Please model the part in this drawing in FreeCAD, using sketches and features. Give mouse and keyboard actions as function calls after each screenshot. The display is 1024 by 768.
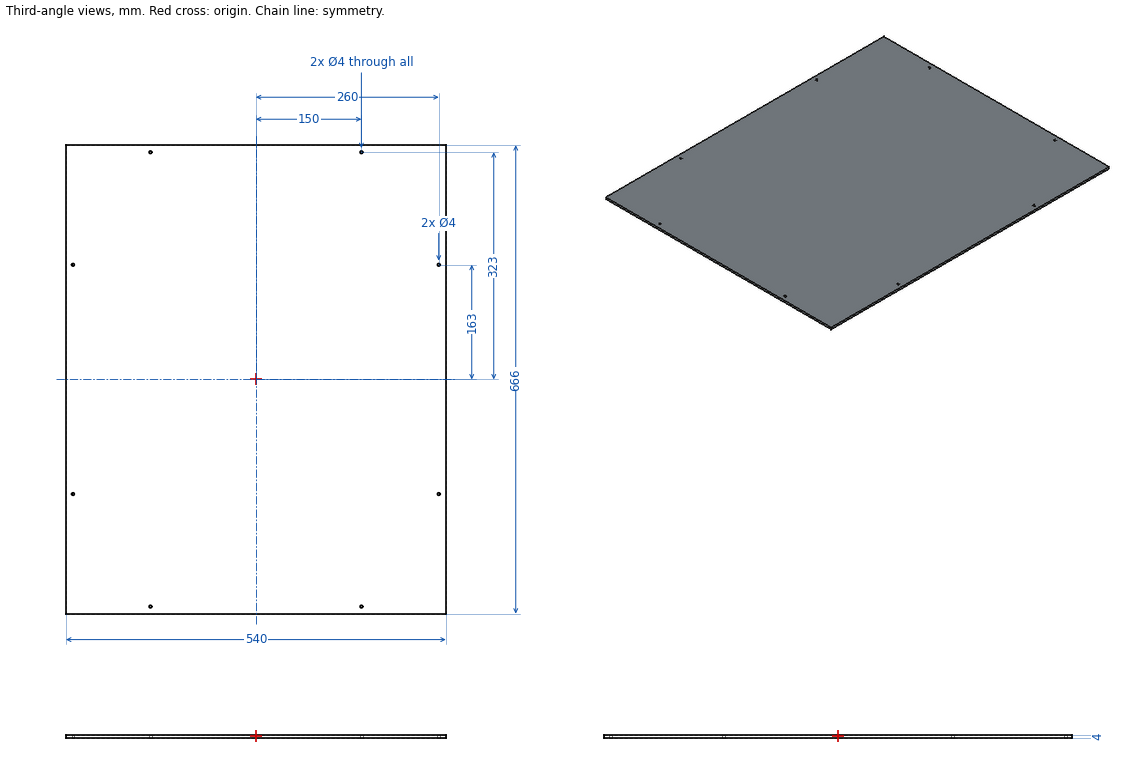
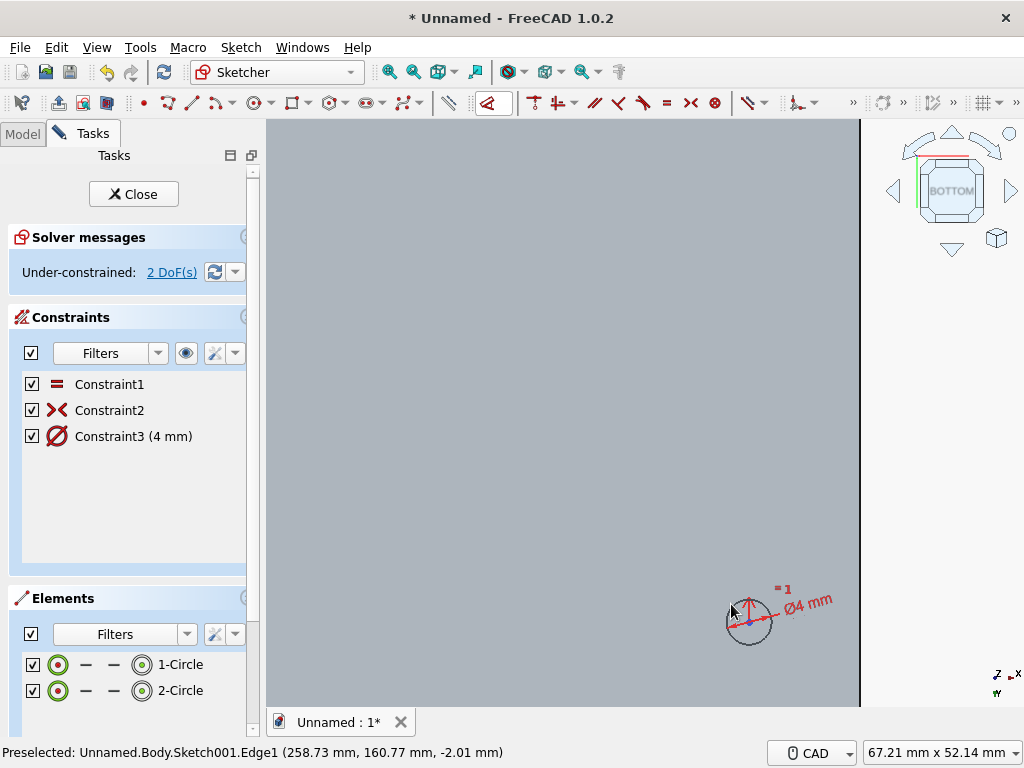
scroll(736, 615, down, 11)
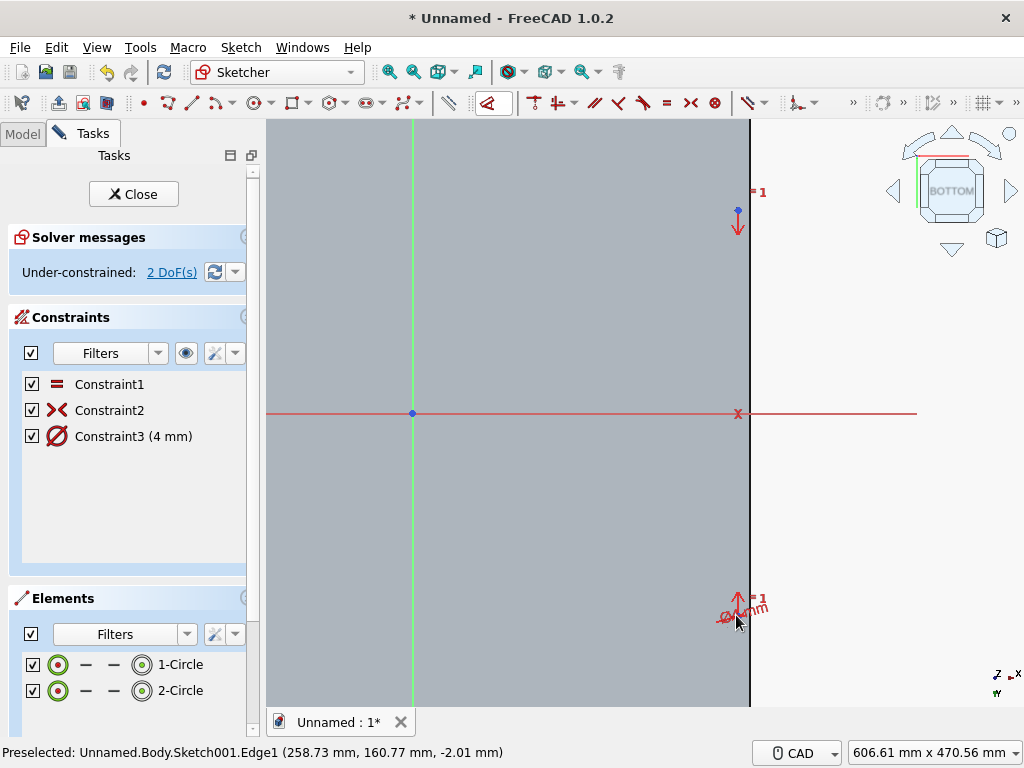
click(738, 617)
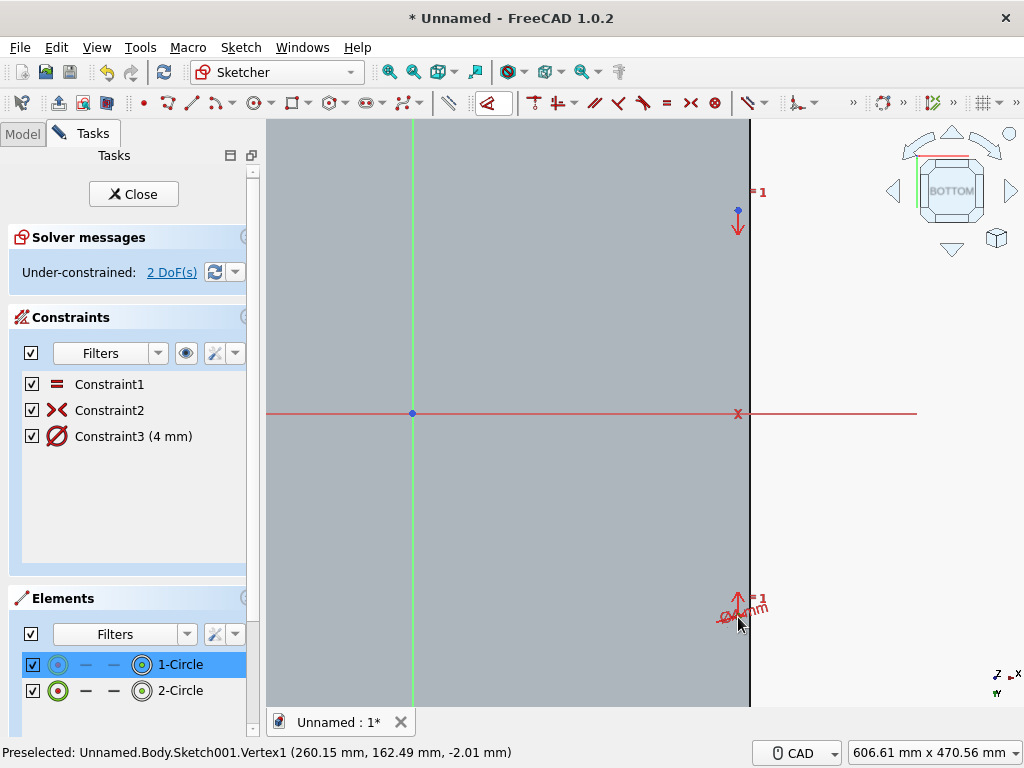
click(506, 104)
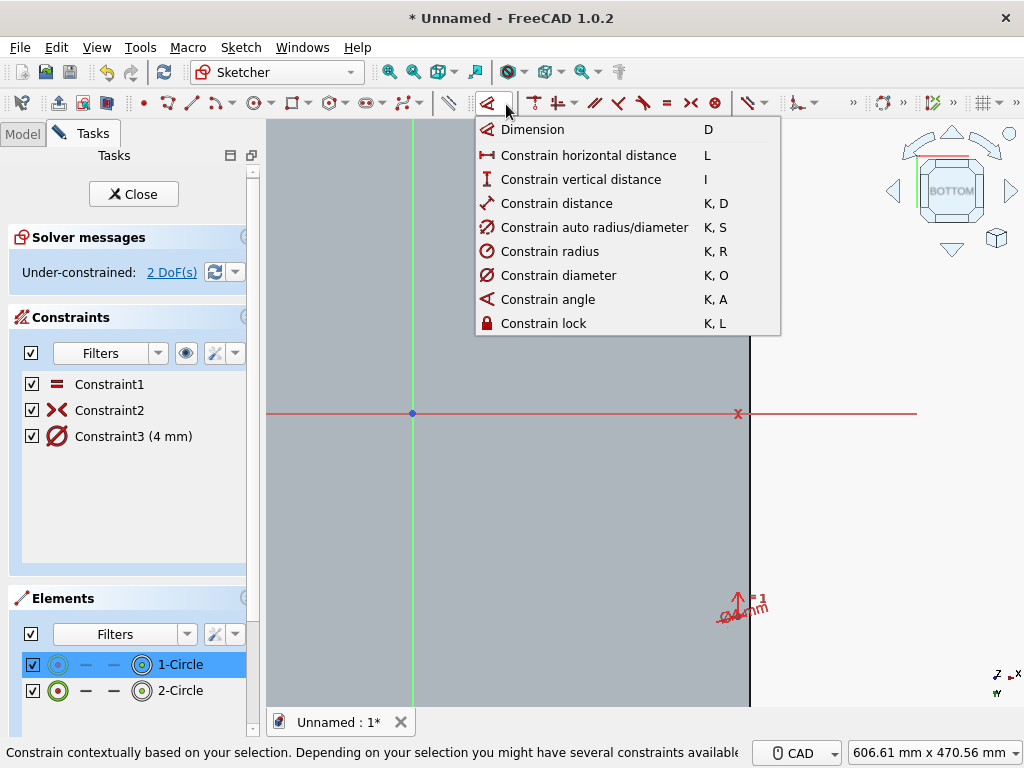
click(628, 155)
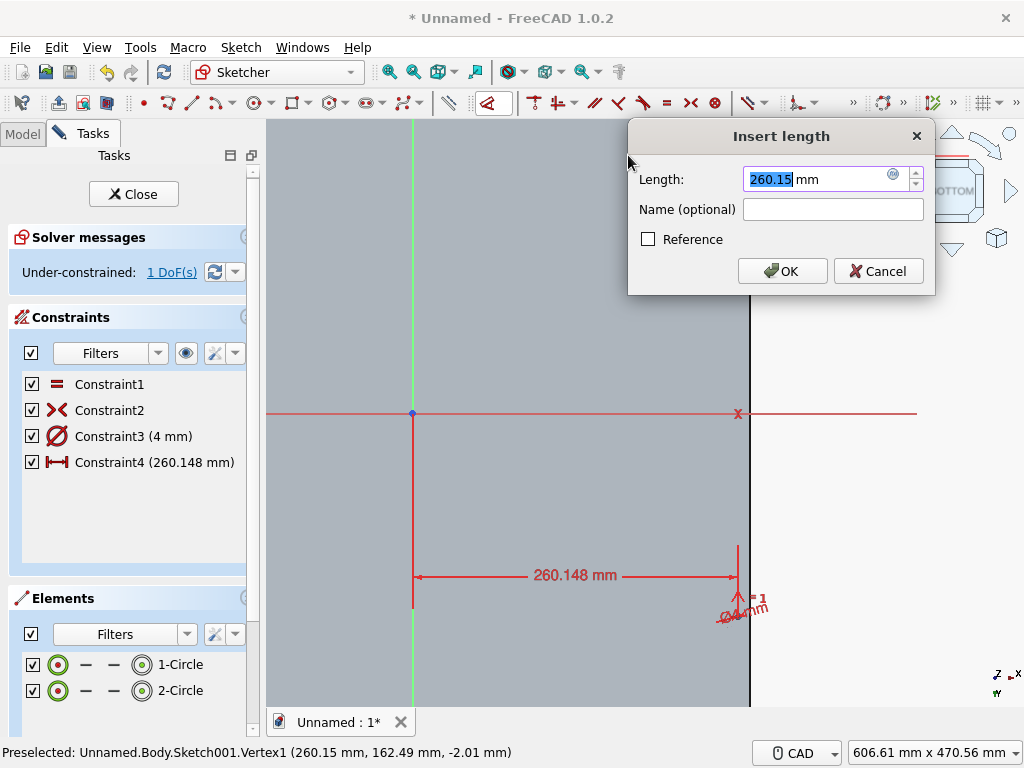
text(260)
key(Return)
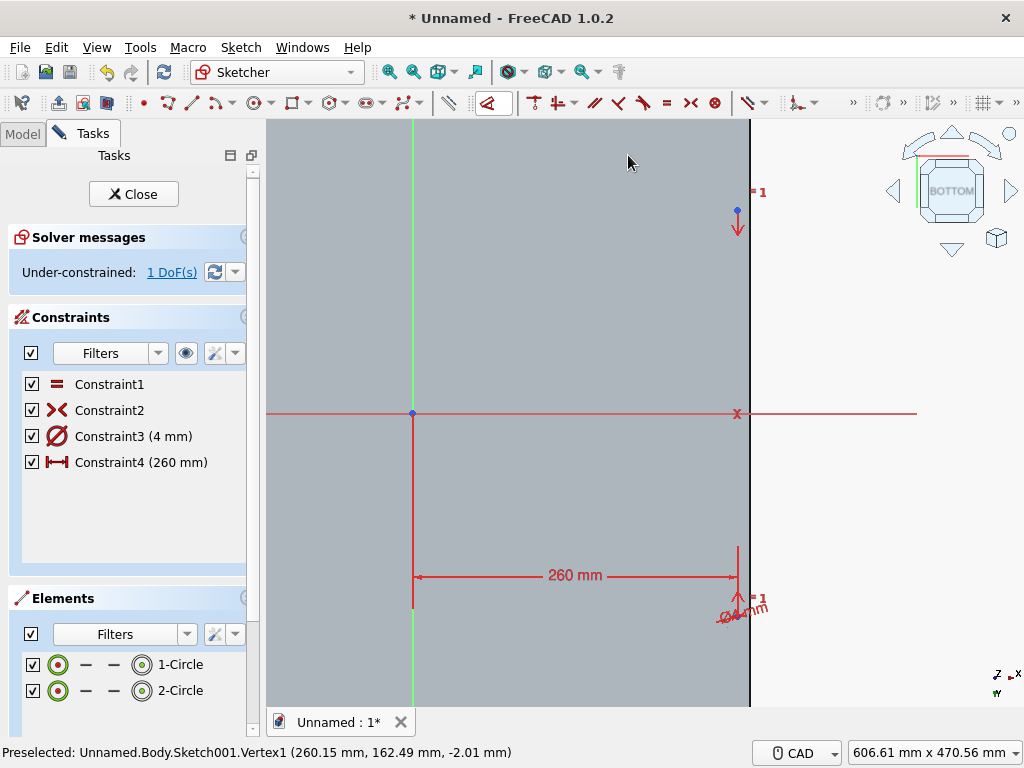
click(738, 617)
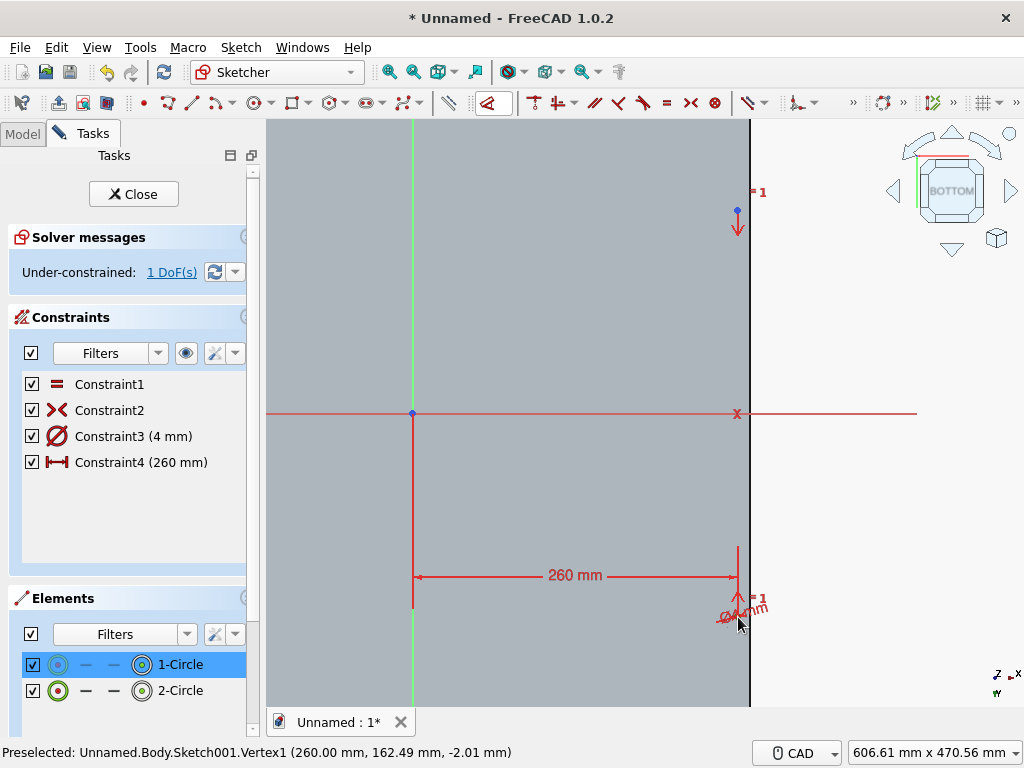
key(i)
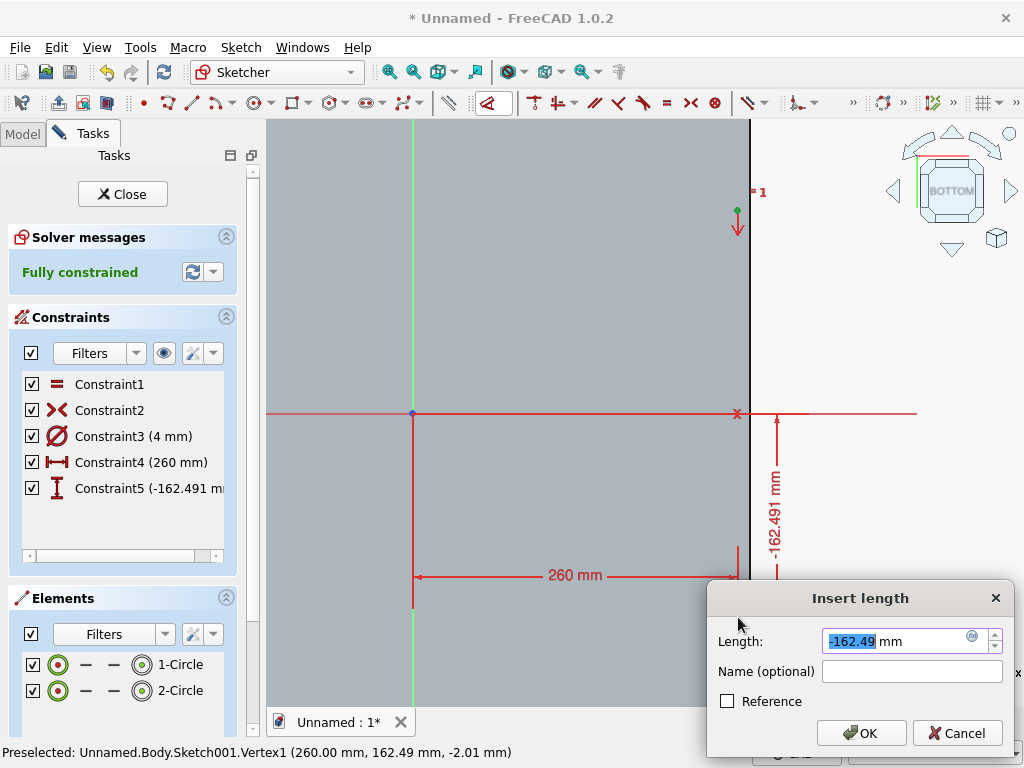
text(-163)
key(Return)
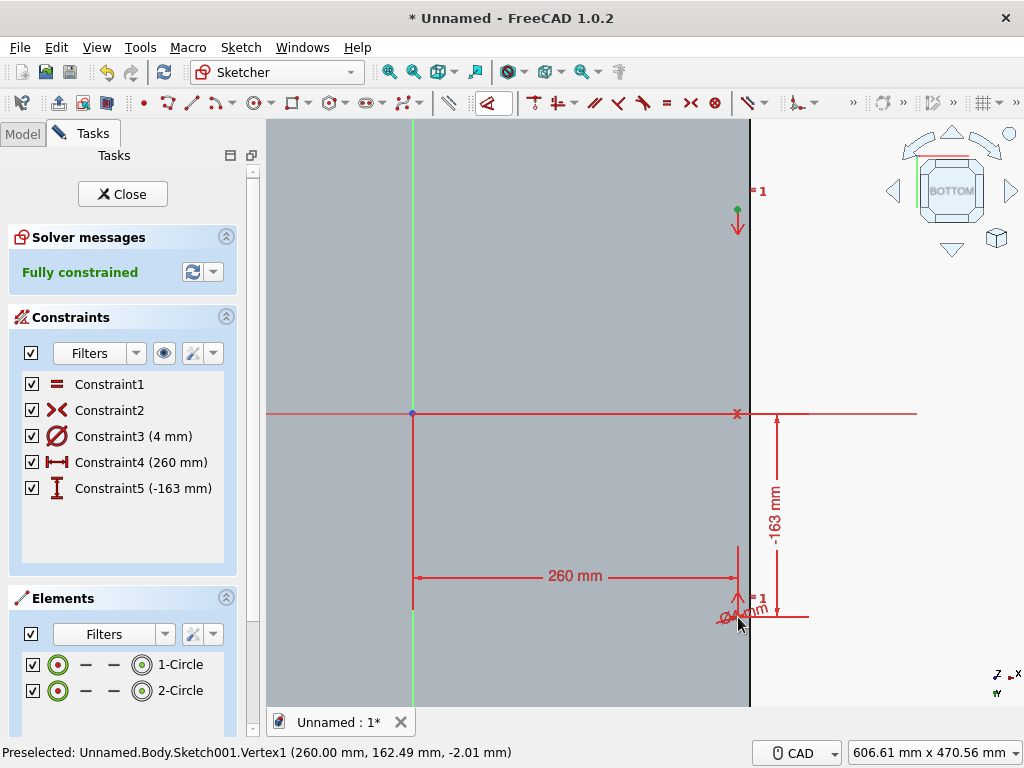
click(123, 194)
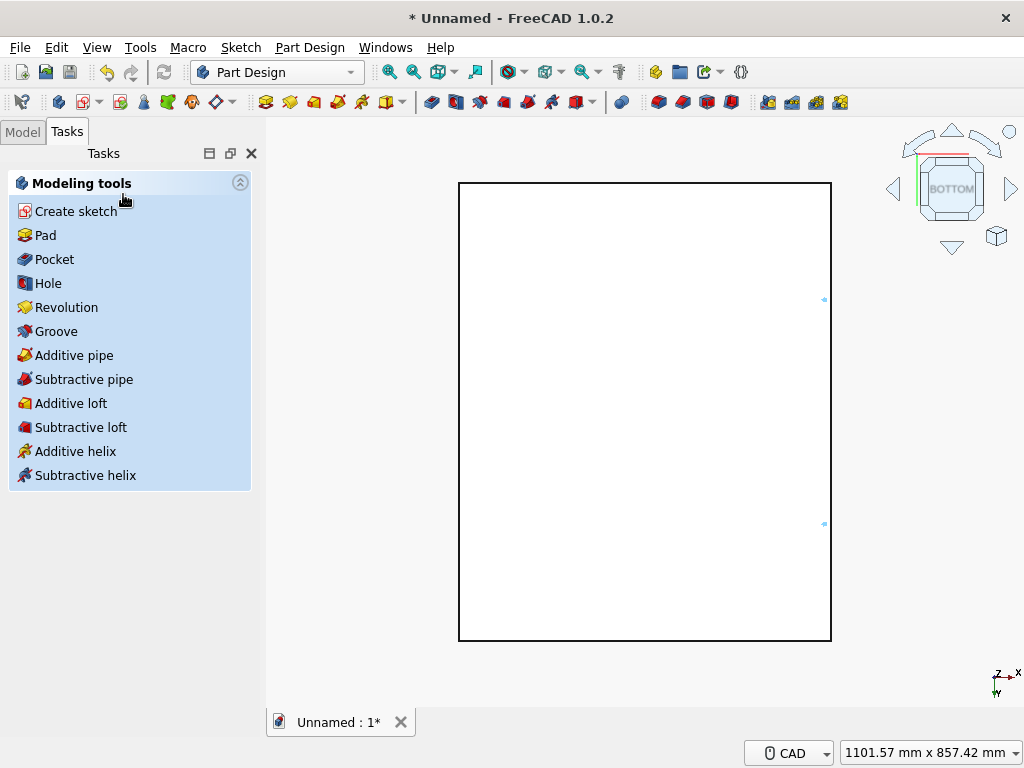
click(432, 102)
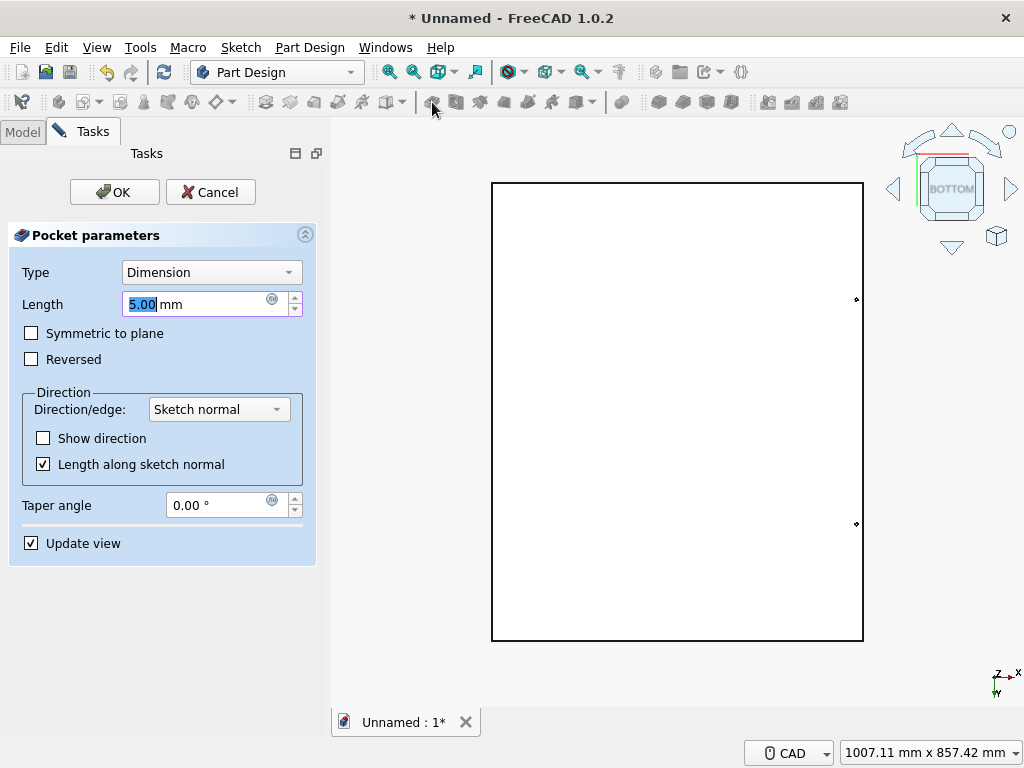
click(212, 272)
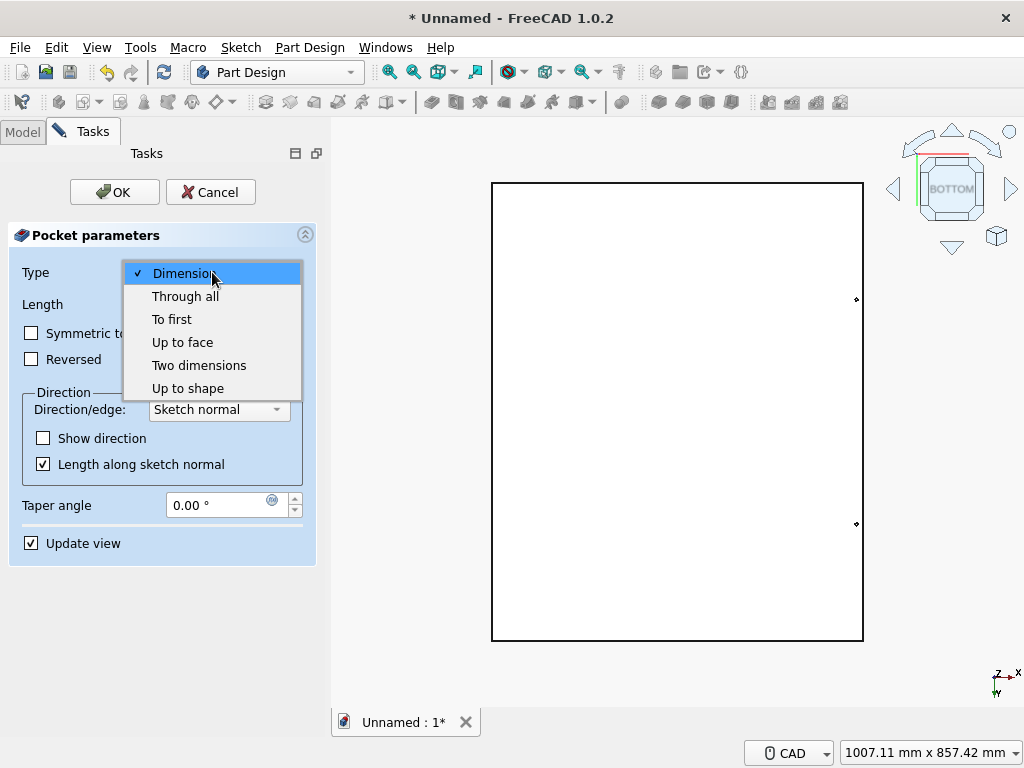
click(212, 296)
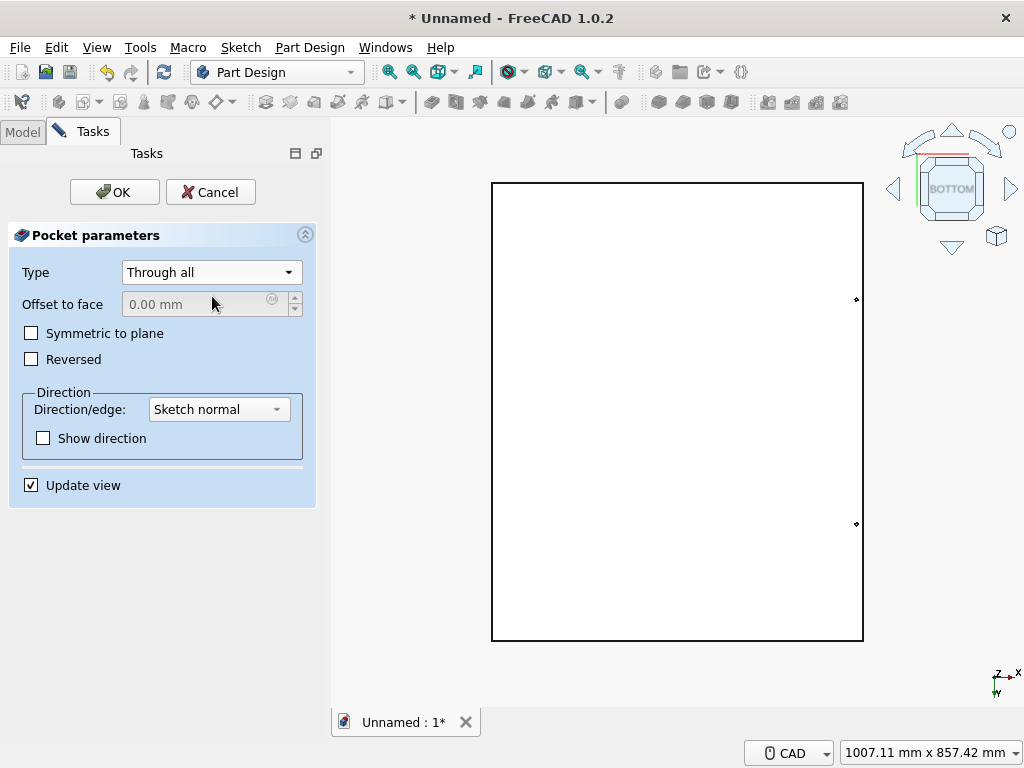
click(115, 192)